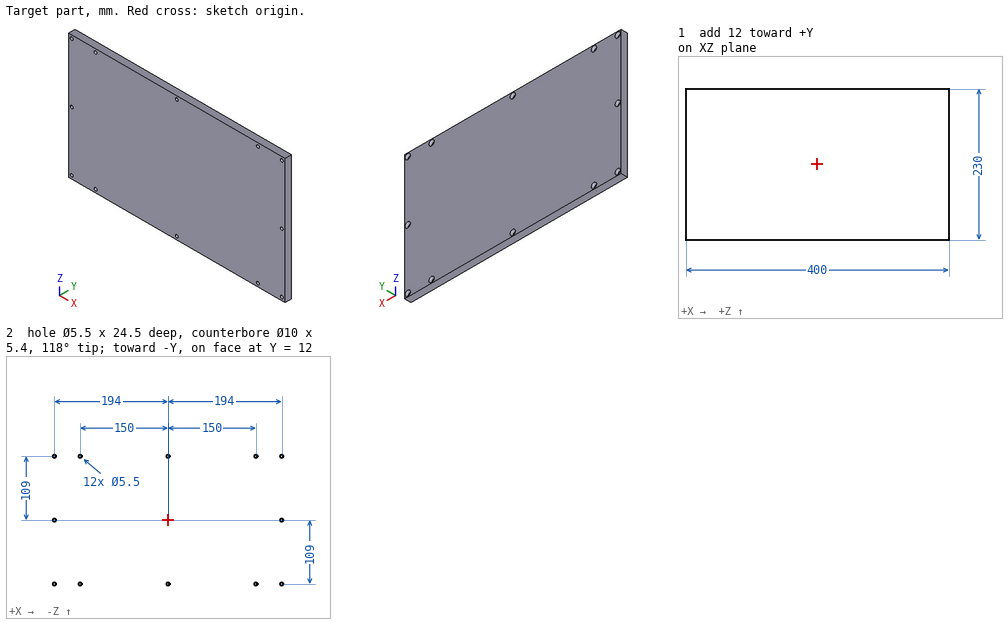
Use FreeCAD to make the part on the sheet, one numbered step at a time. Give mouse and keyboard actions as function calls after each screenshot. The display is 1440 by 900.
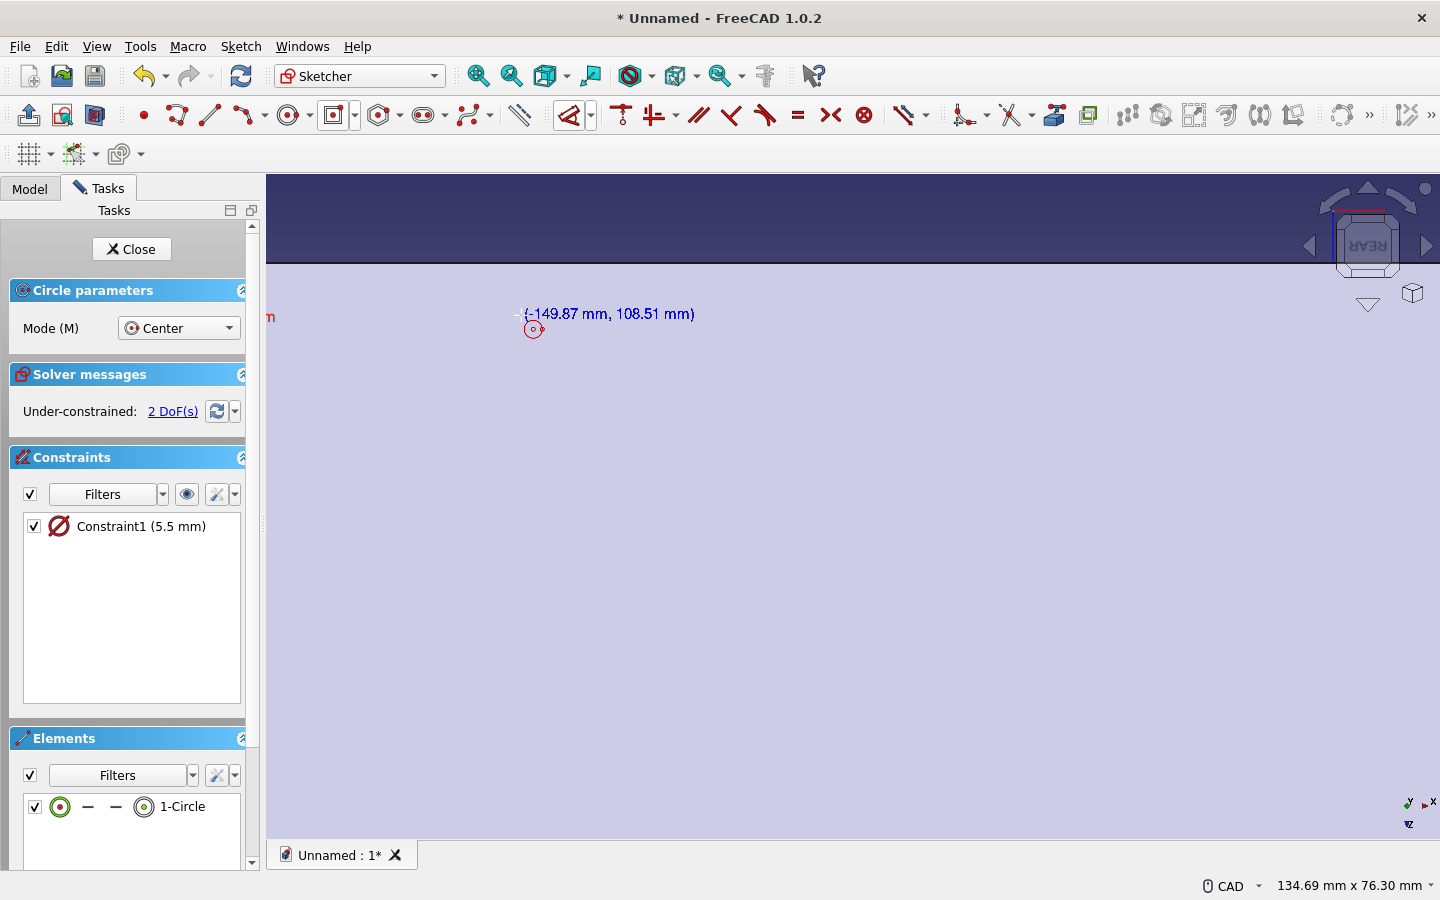
scroll(521, 315, down, 8)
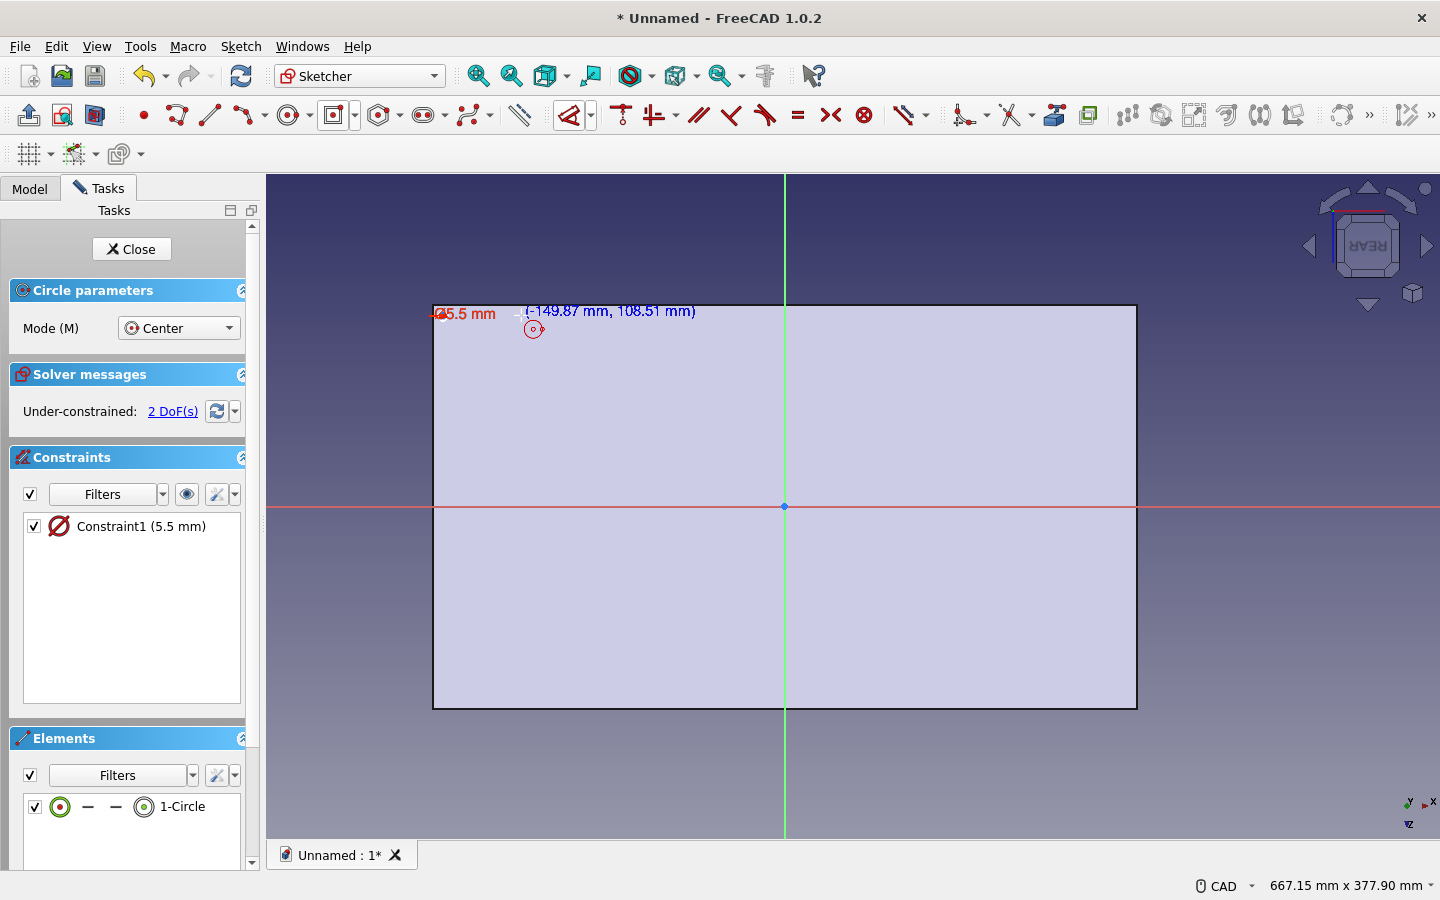
click(521, 315)
move(524, 312)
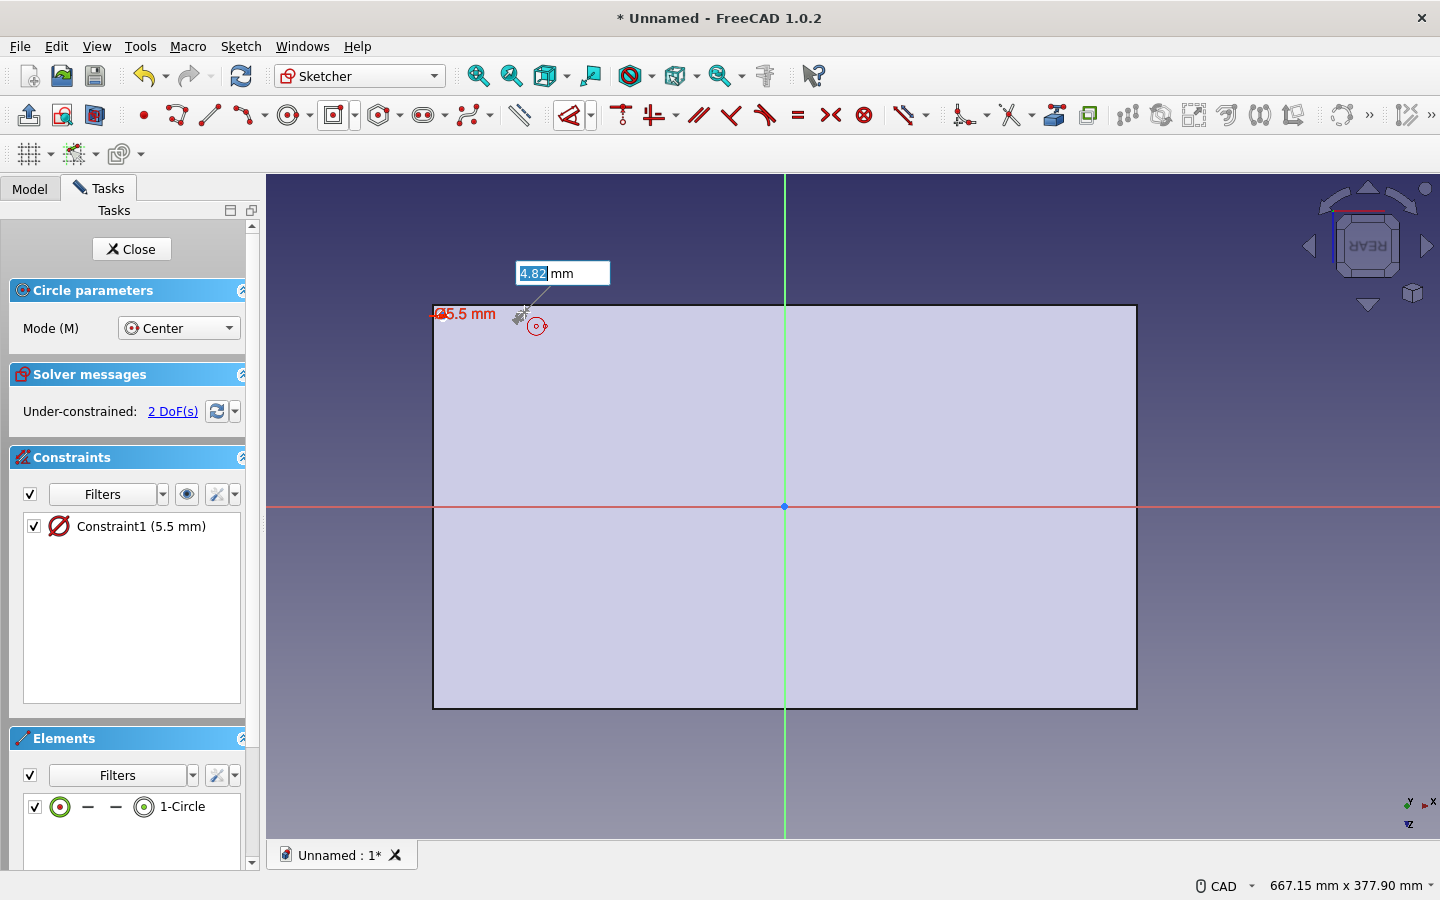
text(5.5)
key(Return)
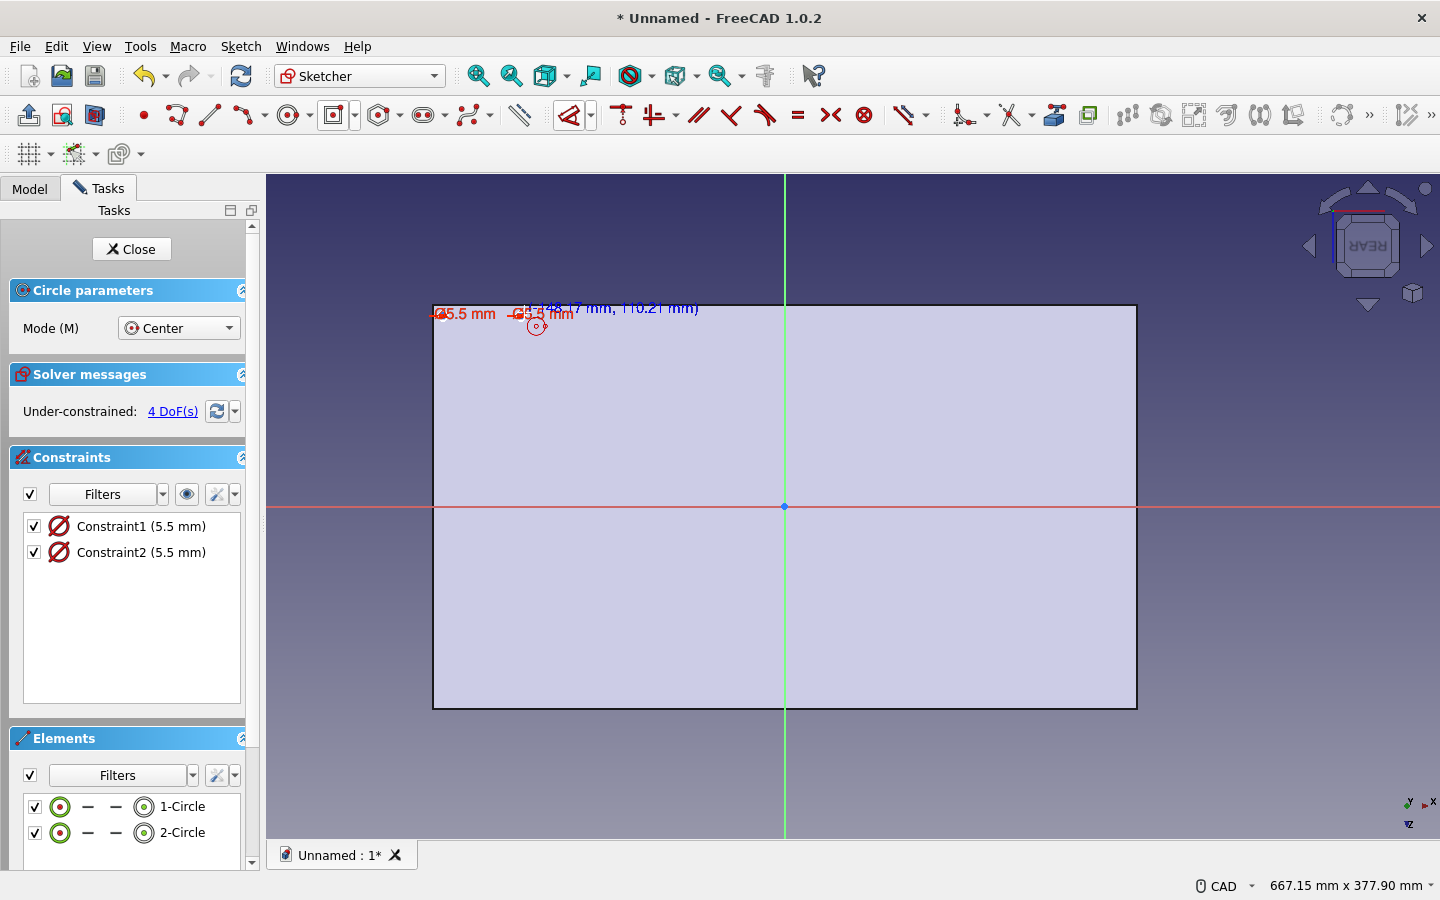
scroll(1049, 315, up, 8)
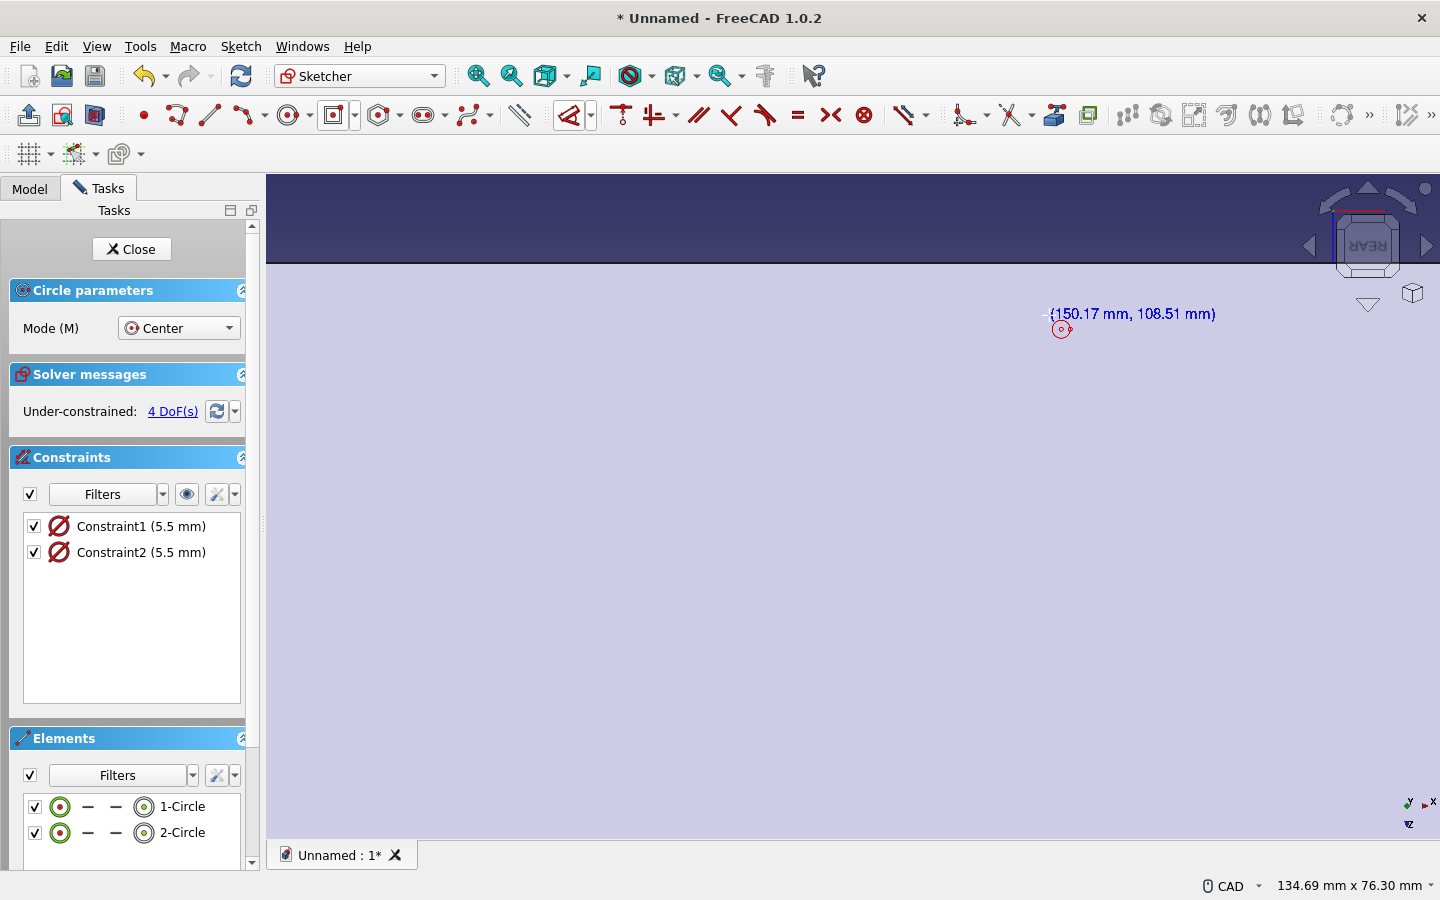
scroll(1049, 315, down, 8)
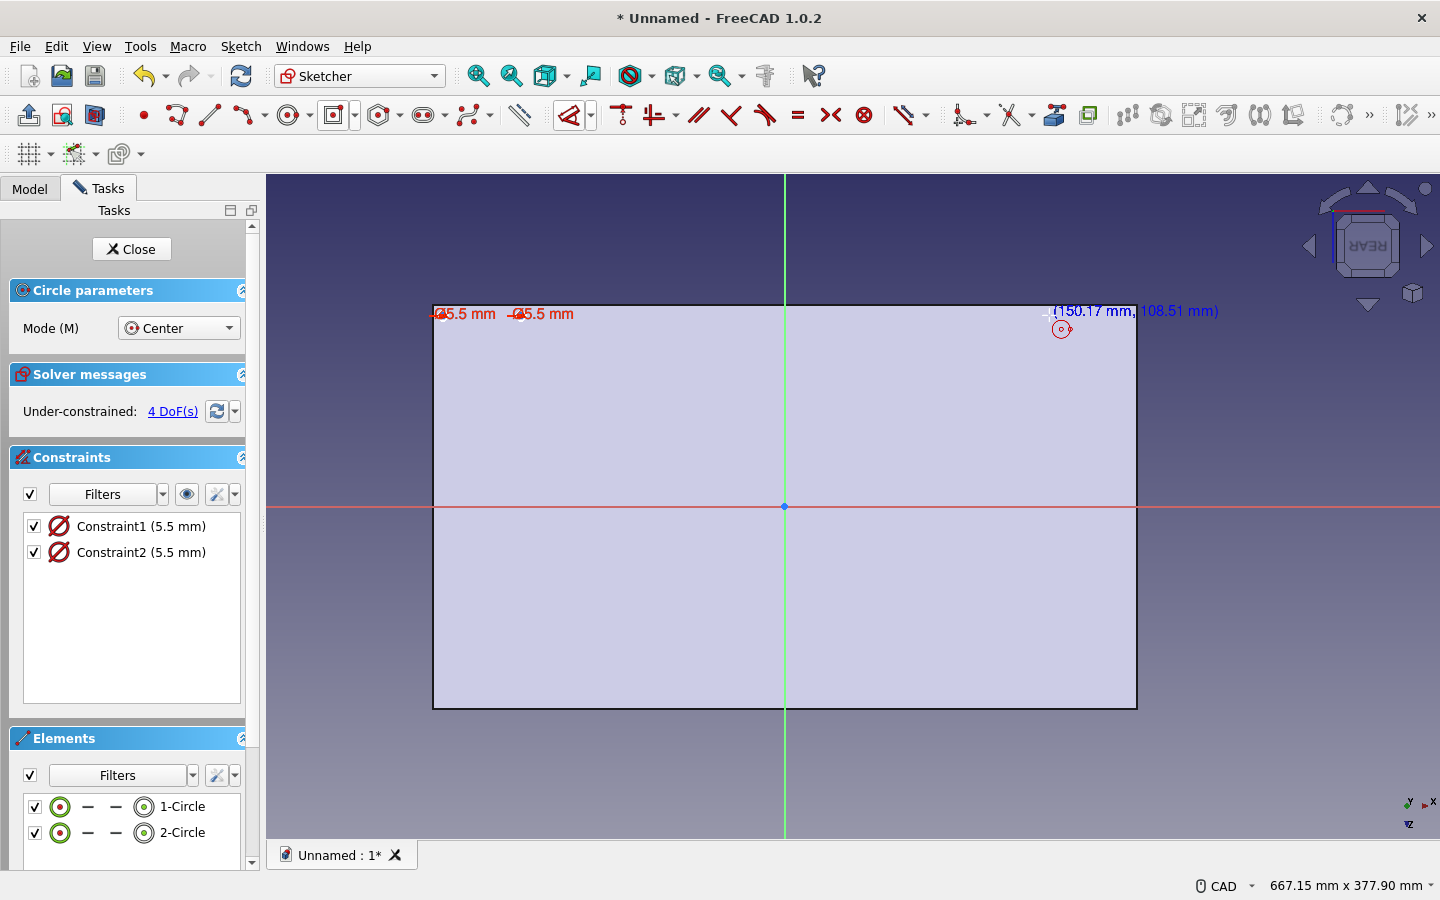
click(1049, 315)
move(1052, 312)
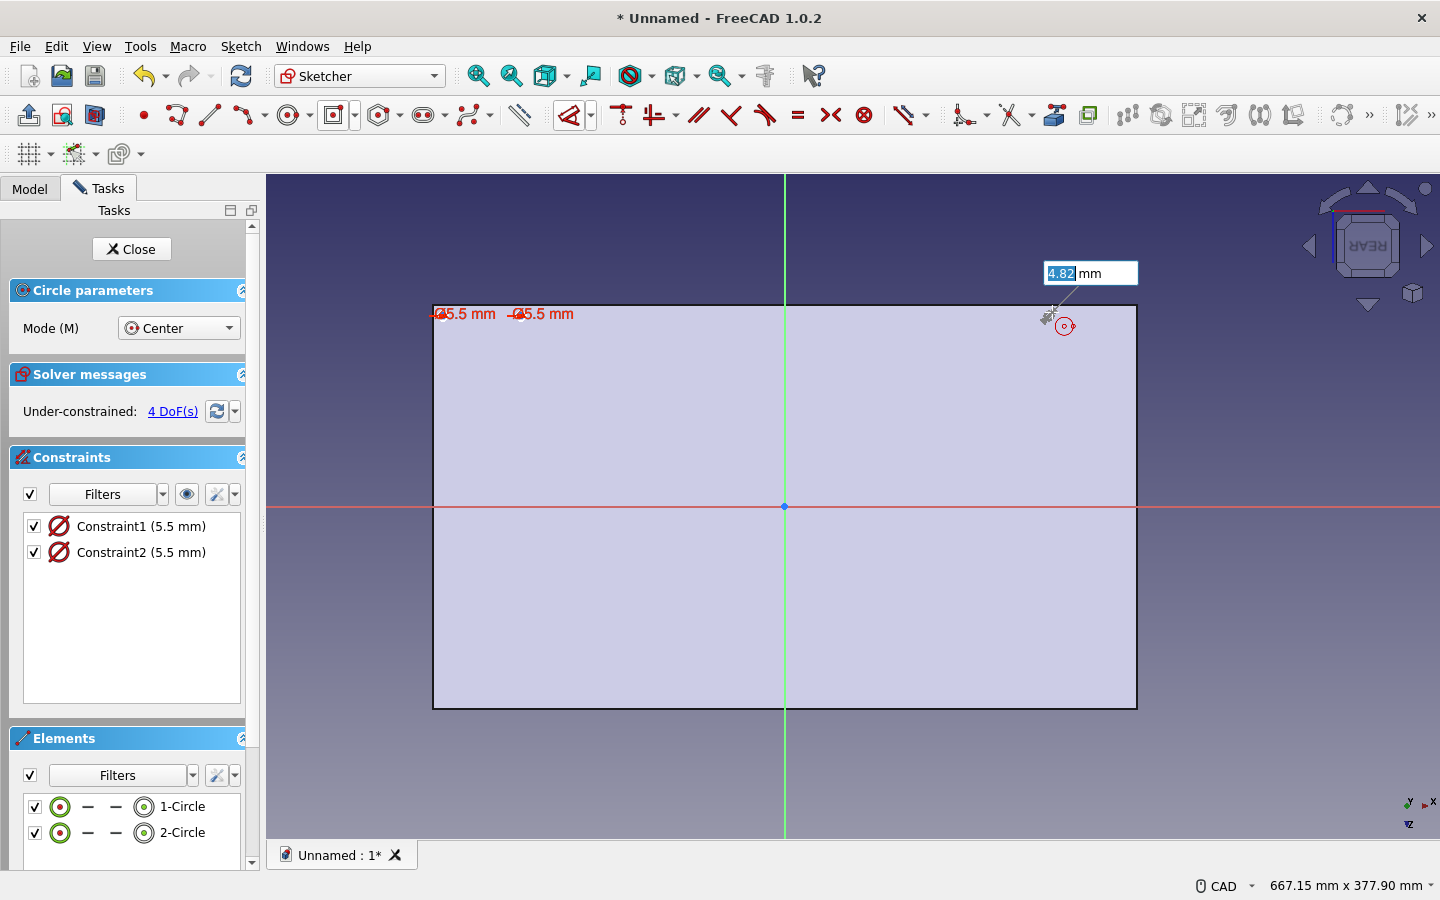
text(5.5)
key(Return)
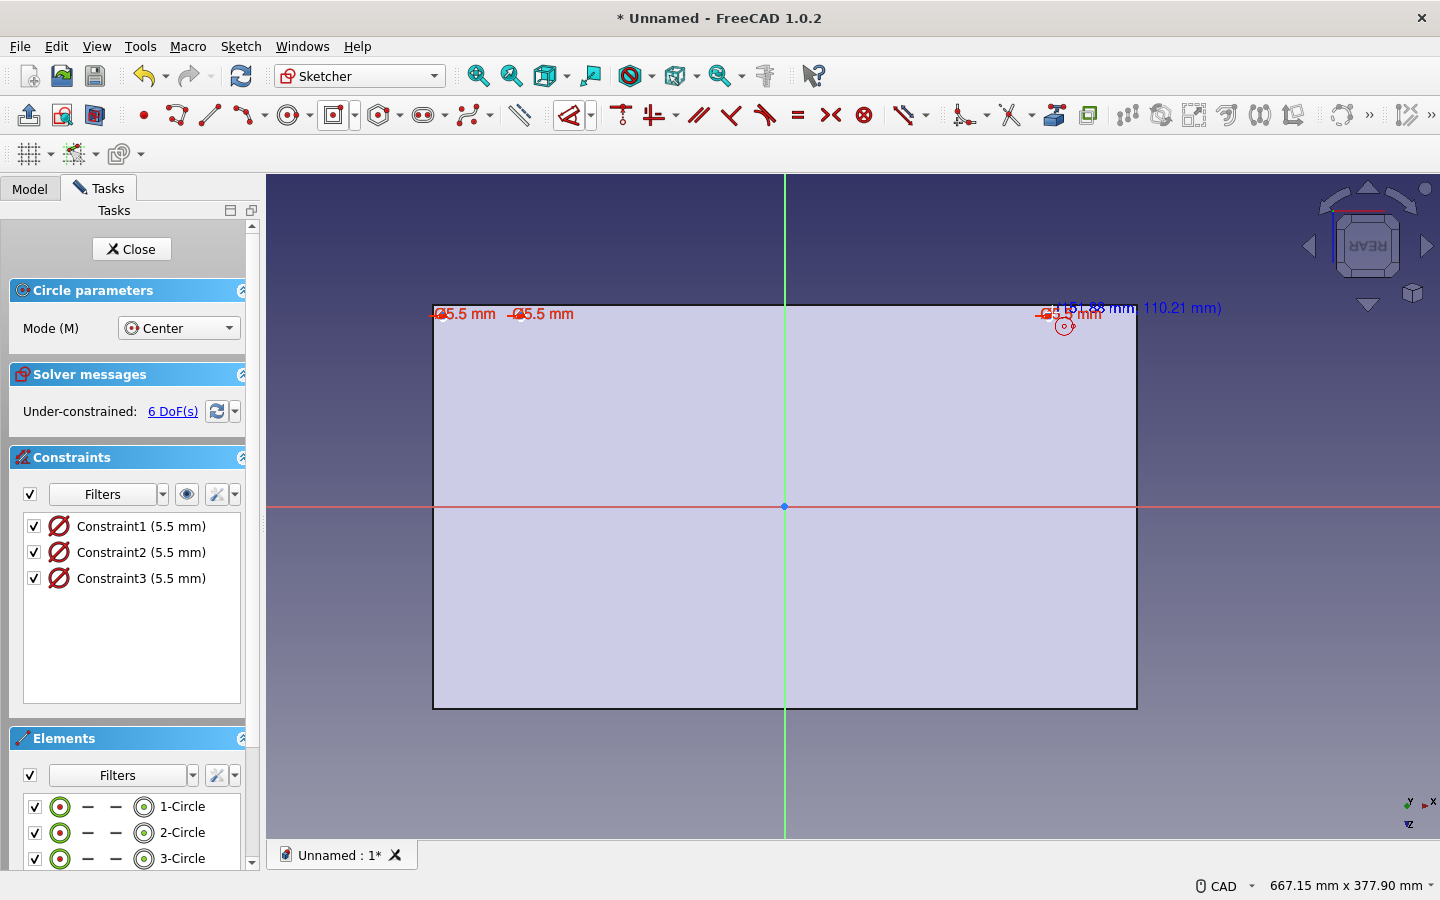
scroll(1126, 315, up, 8)